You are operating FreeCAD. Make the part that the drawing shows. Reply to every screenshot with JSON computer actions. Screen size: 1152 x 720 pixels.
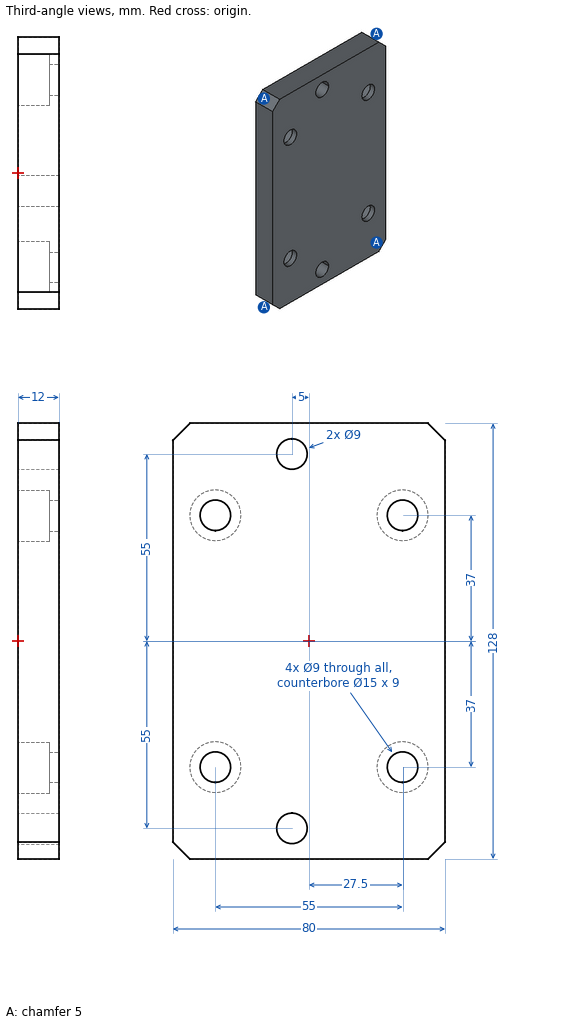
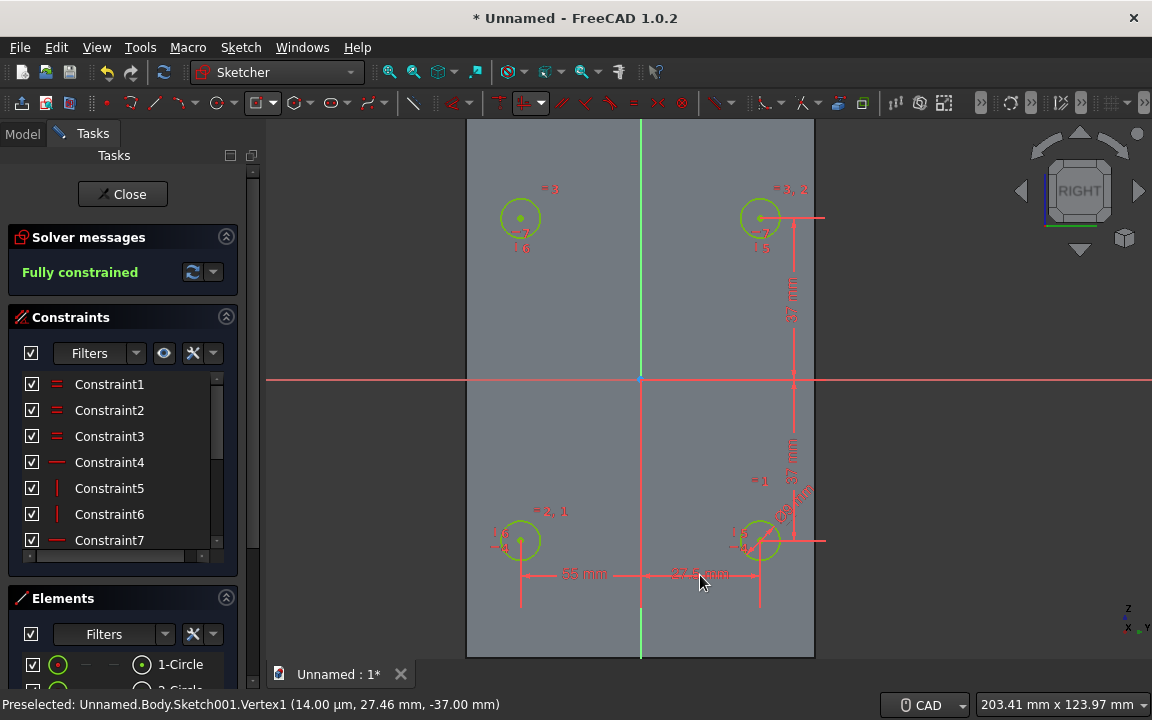
{"action": "left_click", "coordinate": [123, 194]}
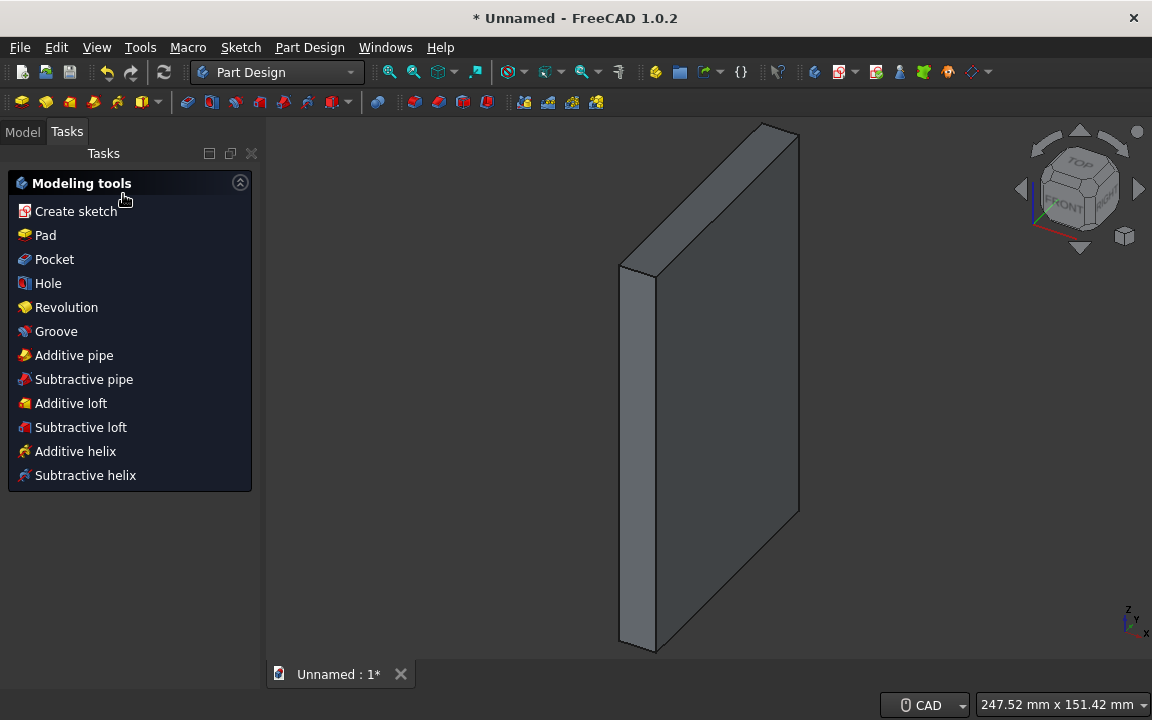
{"action": "left_click", "coordinate": [212, 102]}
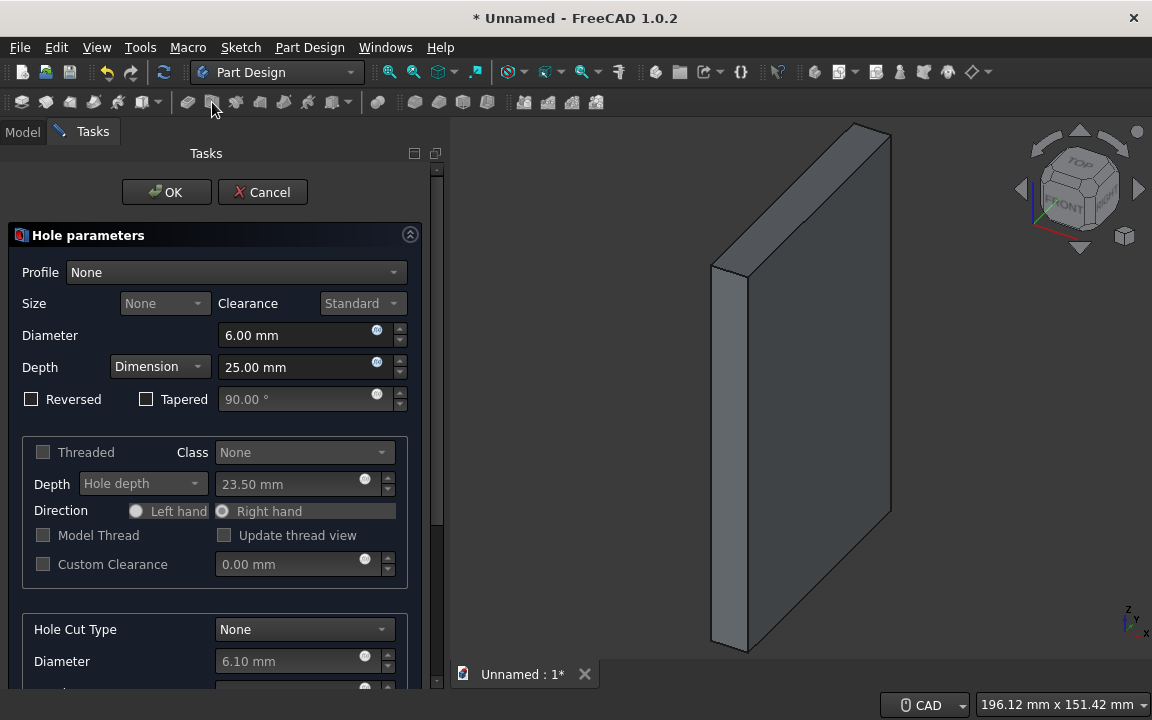
{"action": "triple_click", "coordinate": [305, 335]}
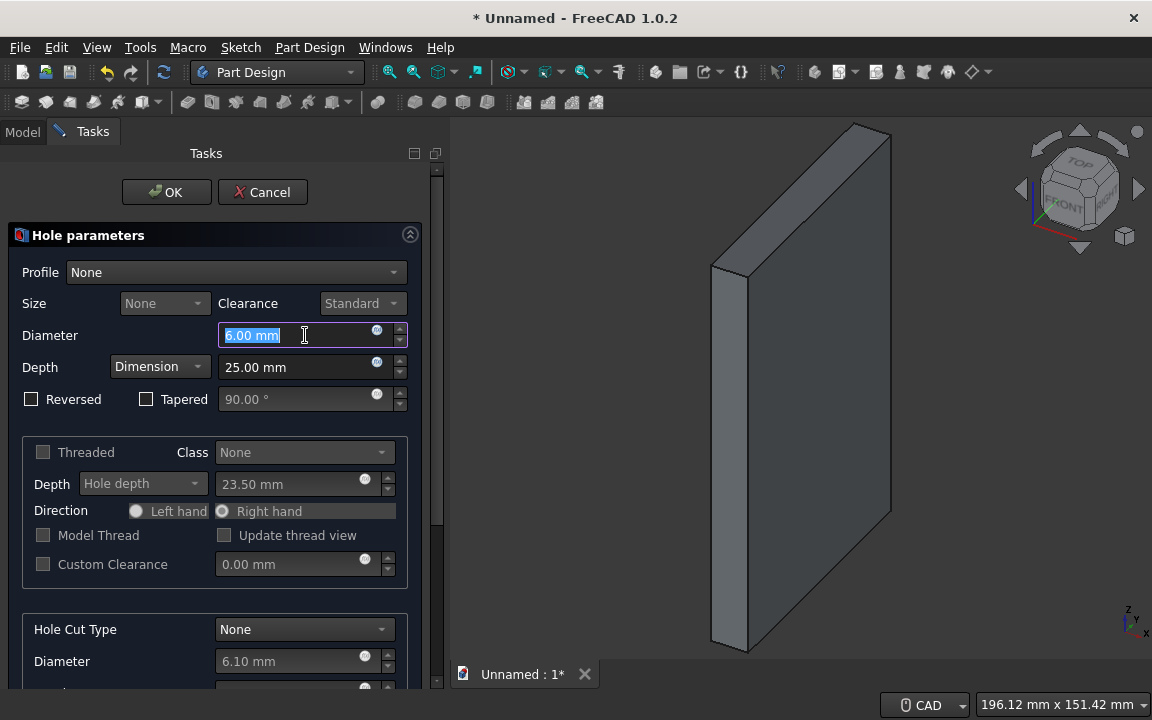
{"action": "type", "text": "9"}
{"action": "key", "text": "Tab"}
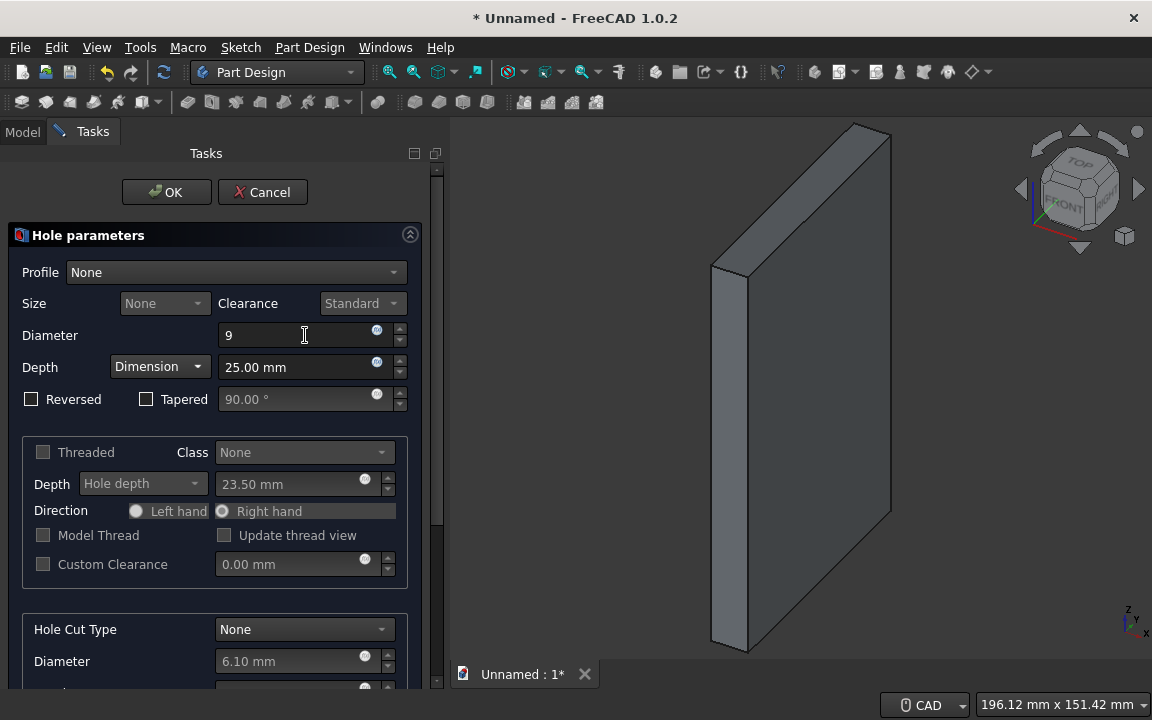
{"action": "left_click", "coordinate": [161, 366]}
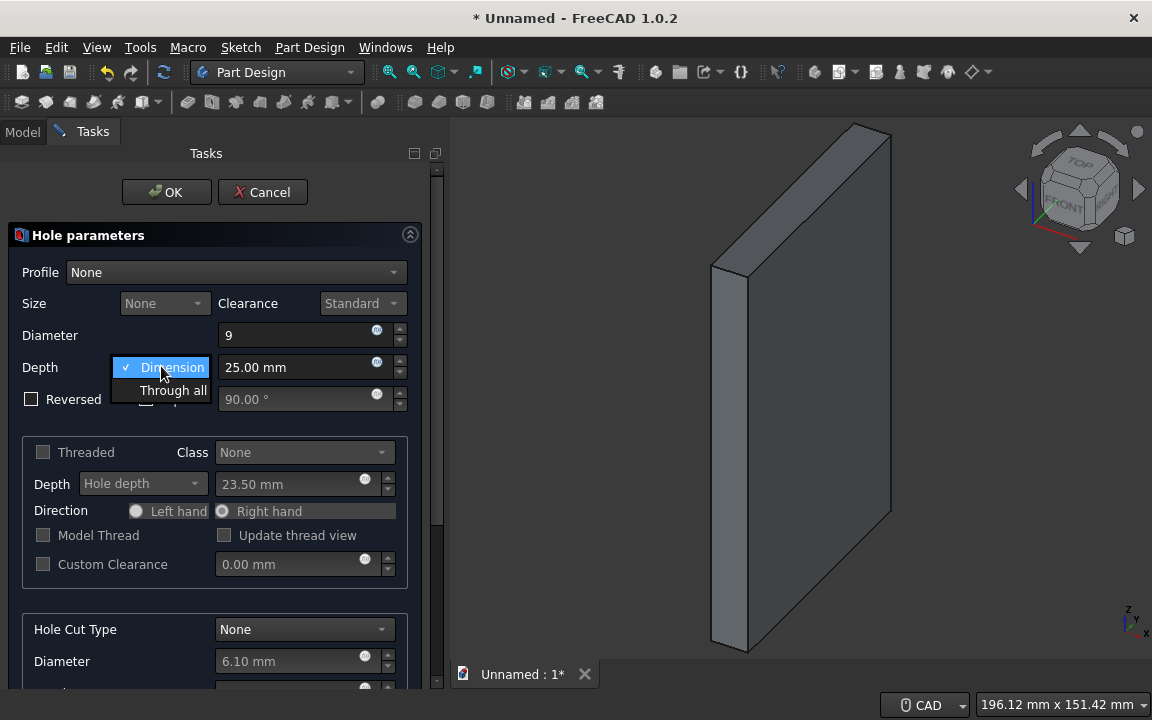
{"action": "left_click", "coordinate": [160, 390]}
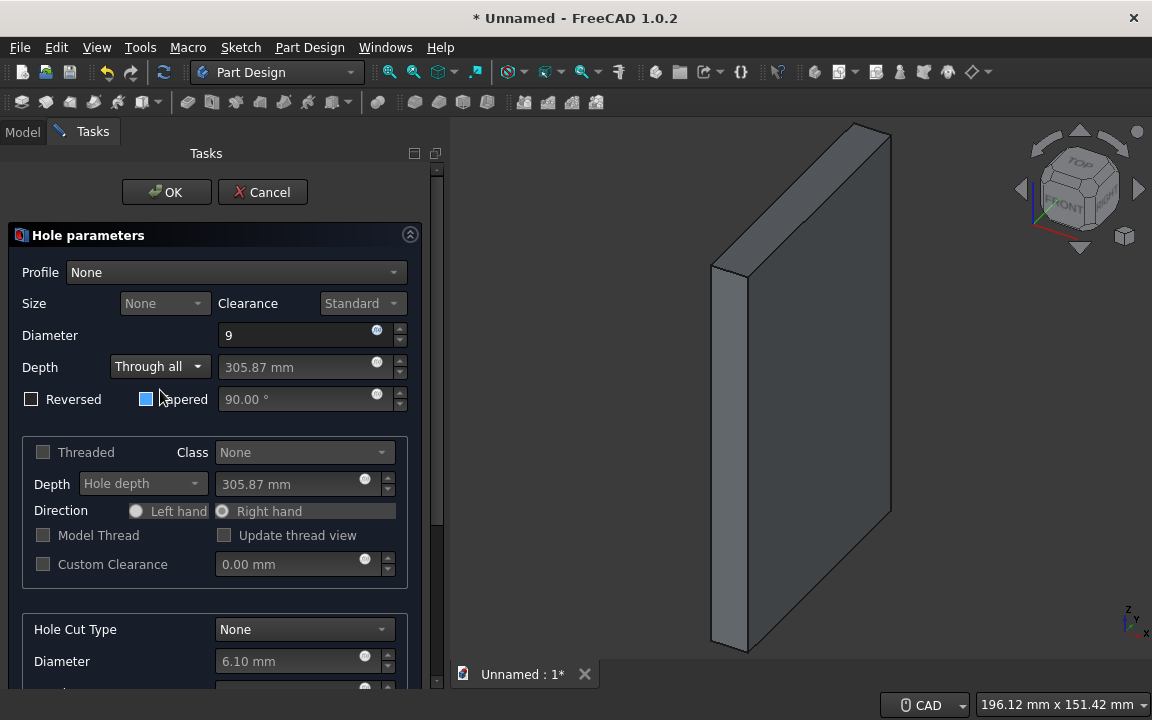
{"action": "left_click", "coordinate": [30, 399]}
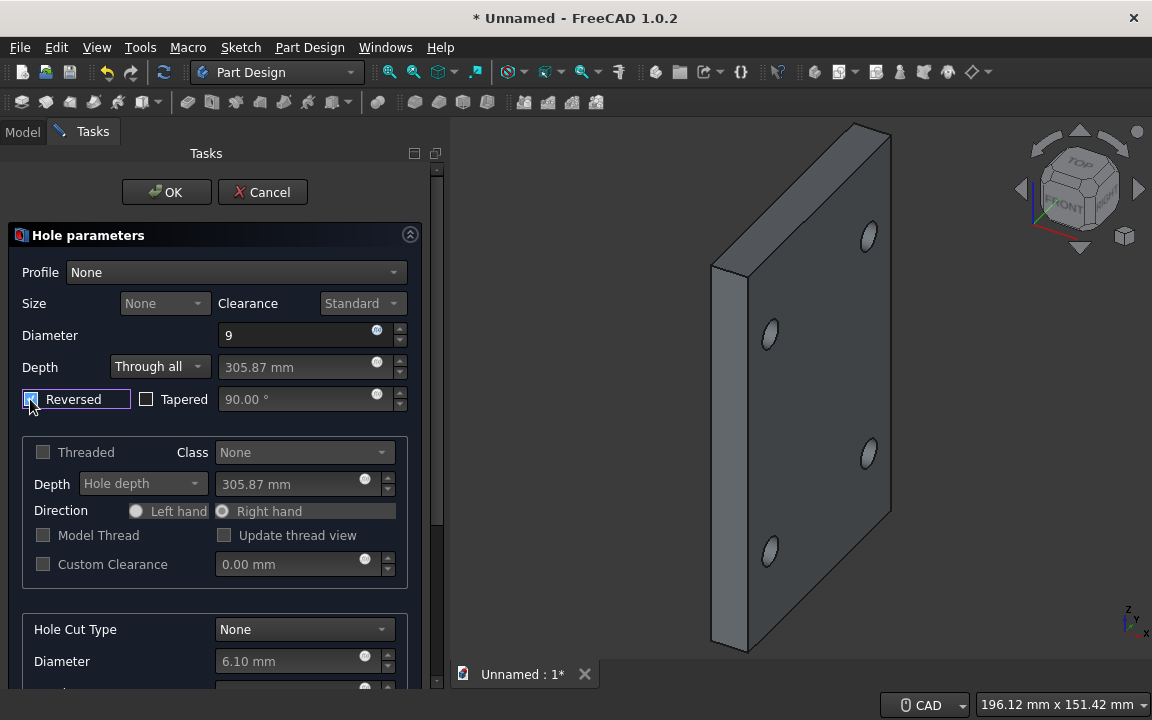
{"action": "left_click", "coordinate": [306, 630]}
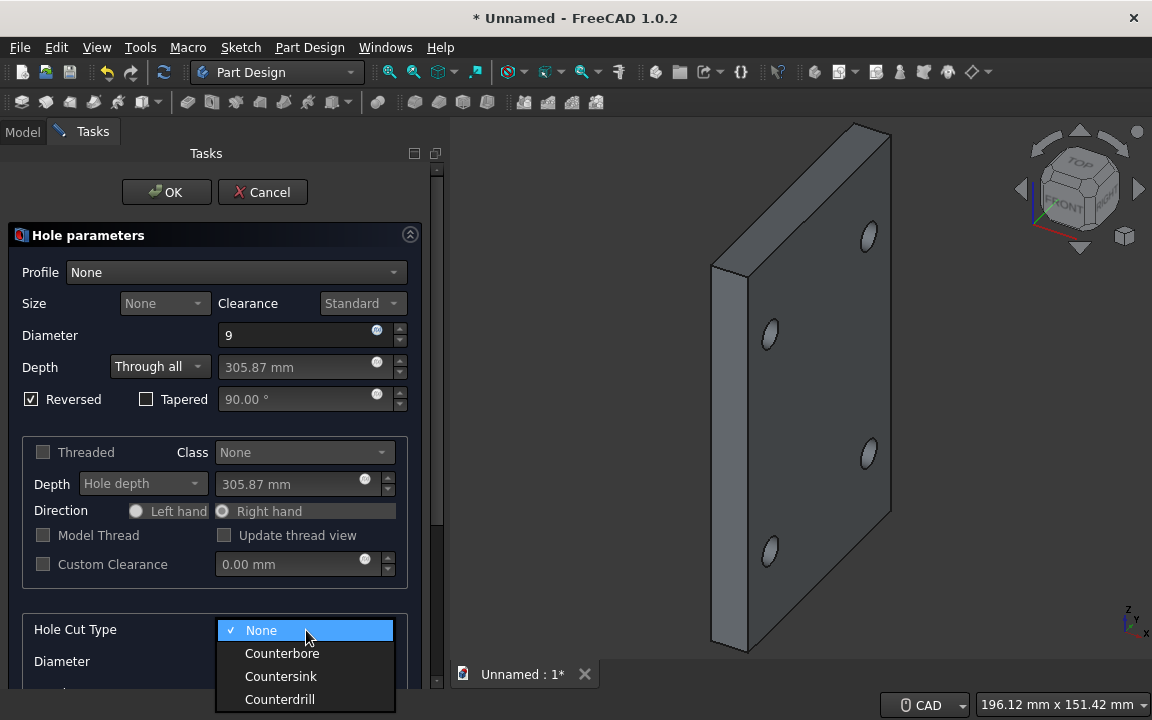
{"action": "left_click", "coordinate": [304, 654]}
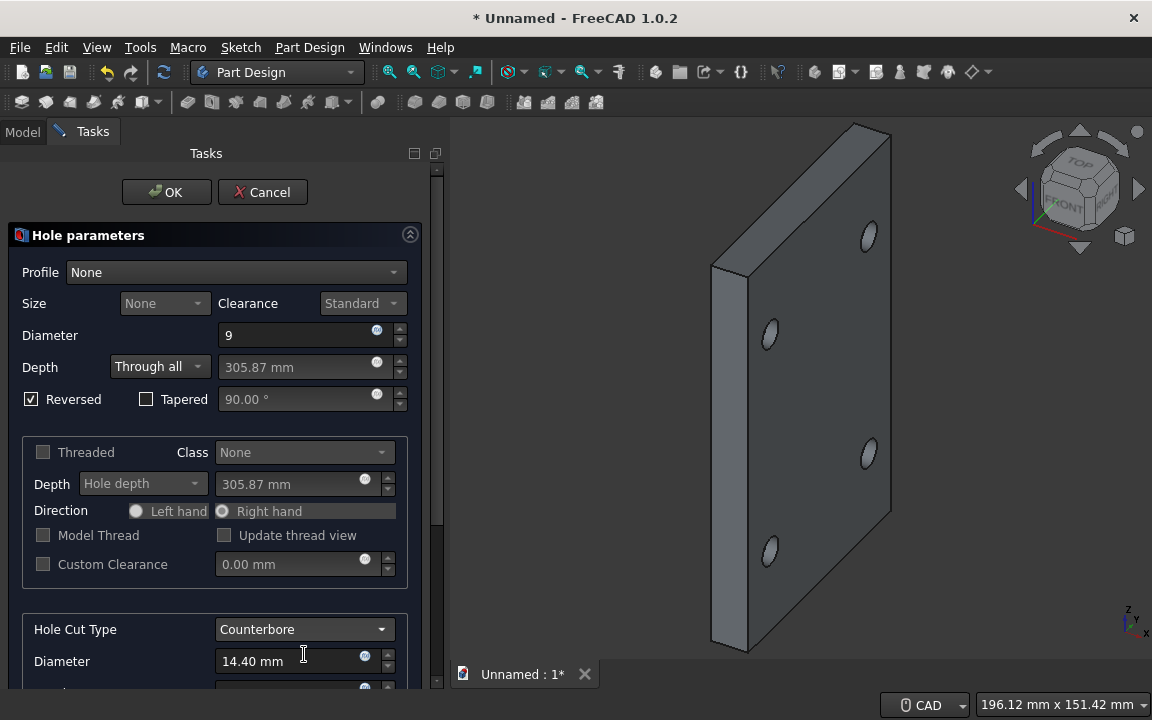
{"action": "triple_click", "coordinate": [298, 661]}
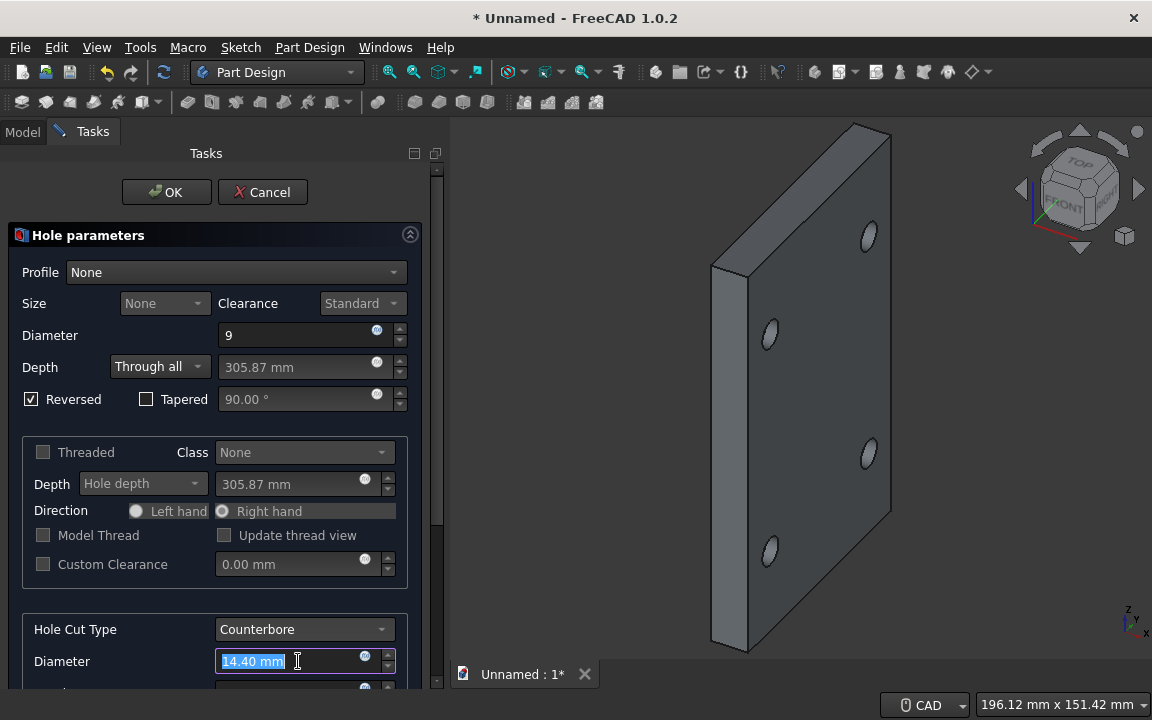
{"action": "type", "text": "15"}
{"action": "key", "text": "Tab"}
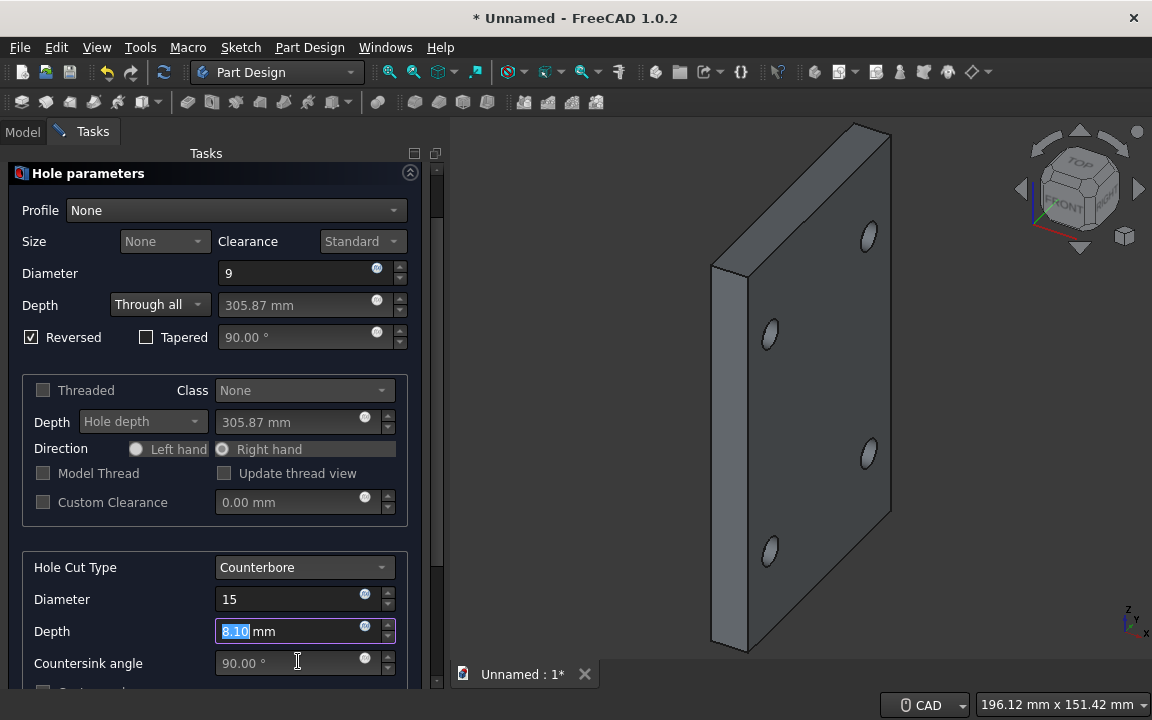
{"action": "type", "text": "9"}
{"action": "key", "text": "Tab"}